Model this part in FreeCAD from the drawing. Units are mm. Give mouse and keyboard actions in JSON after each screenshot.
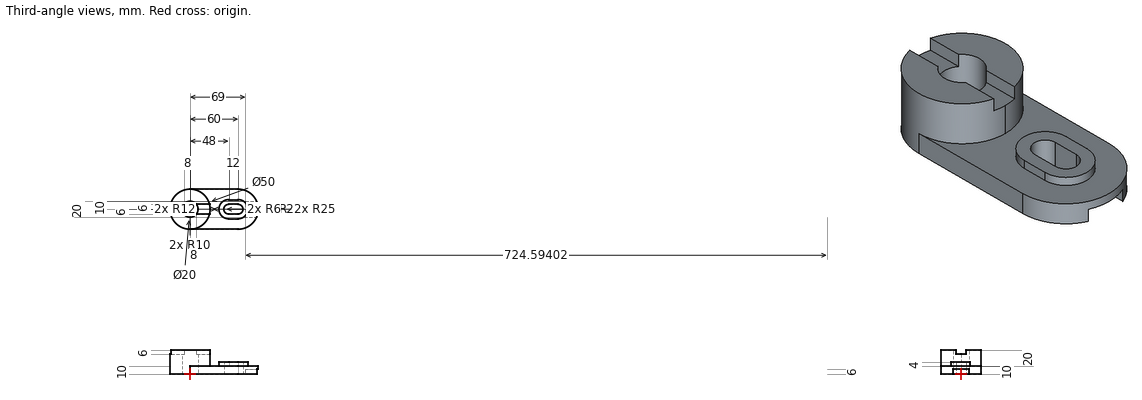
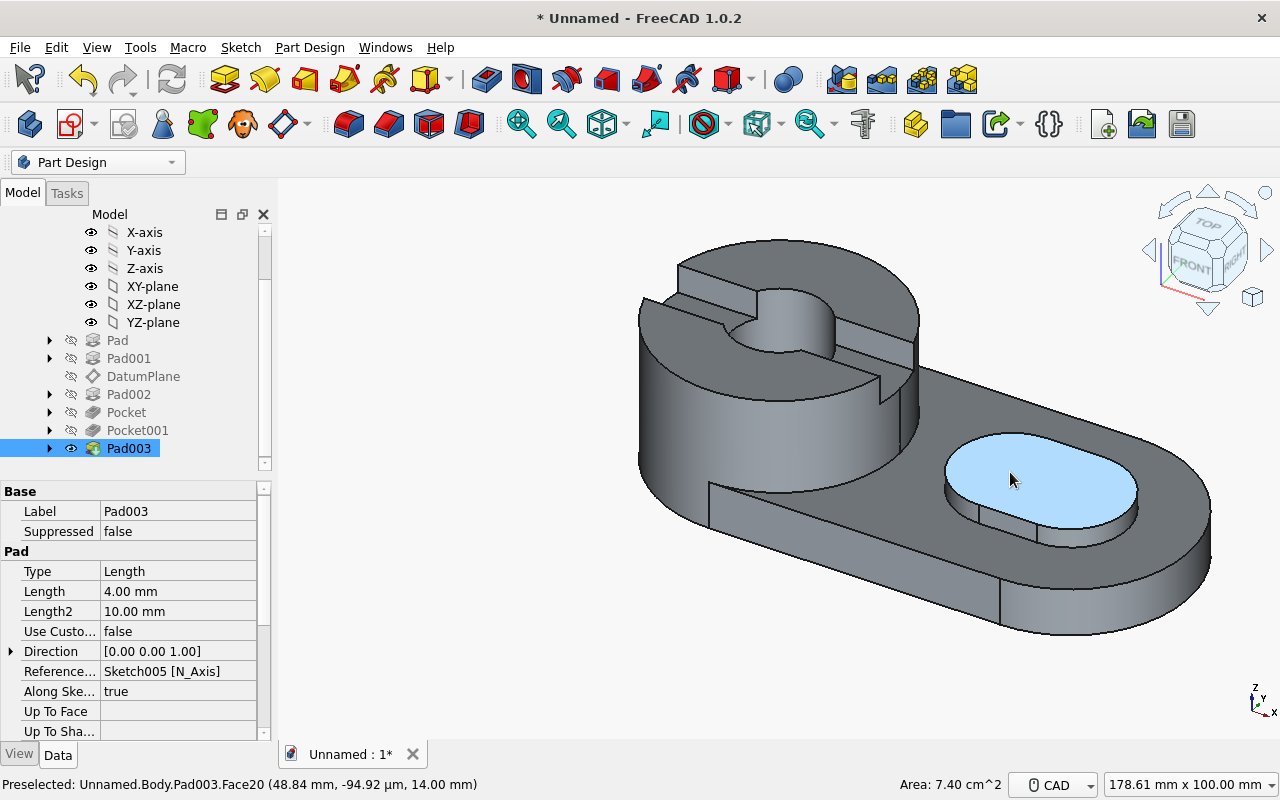
{"action": "left_click", "coordinate": [70, 124]}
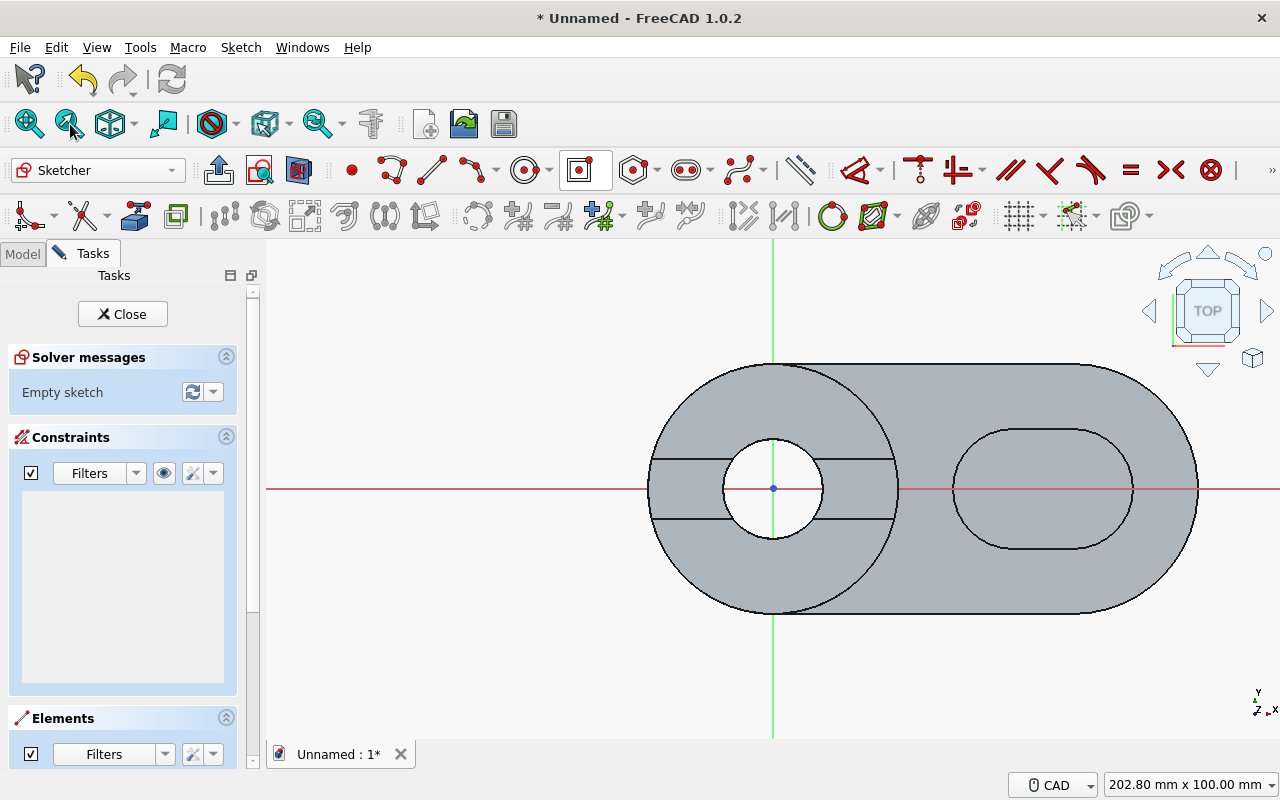
{"action": "left_click", "coordinate": [300, 170]}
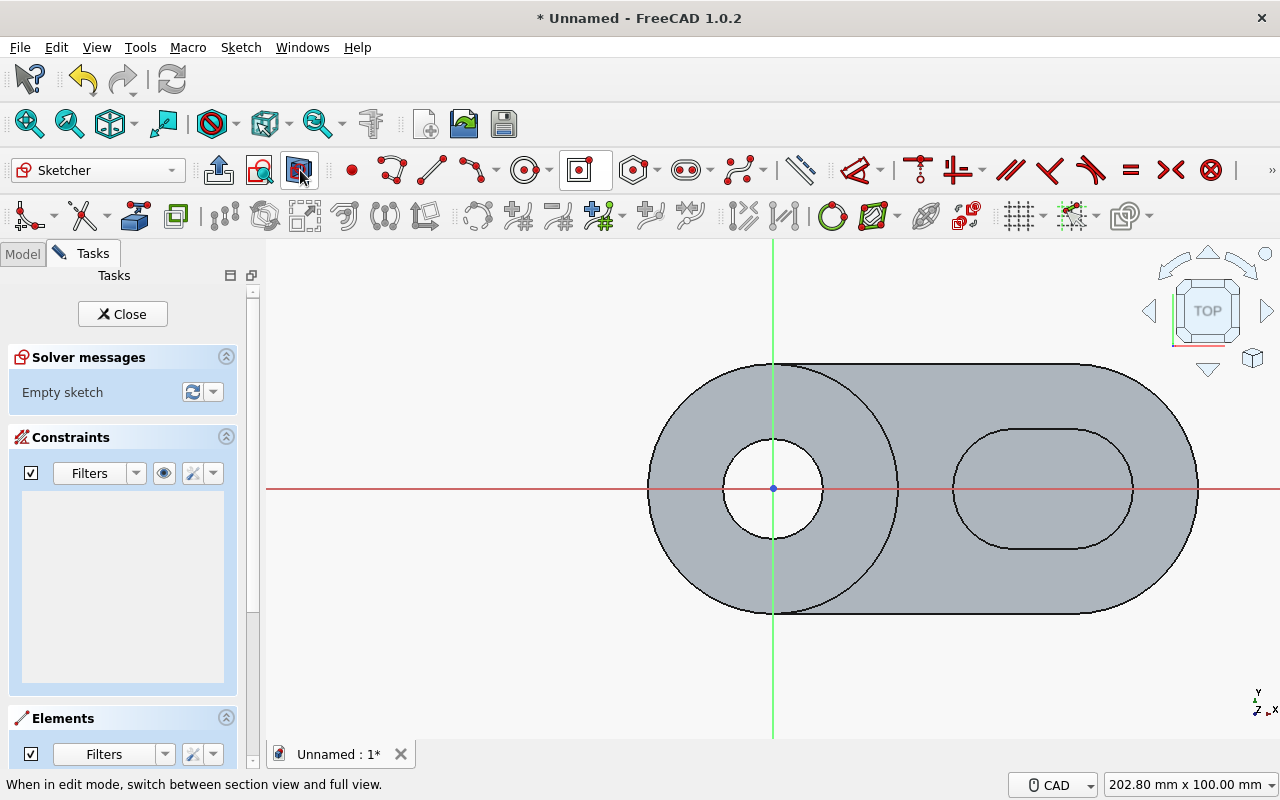
{"action": "scroll", "coordinate": [1115, 489], "scroll_direction": "up", "scroll_amount": 8}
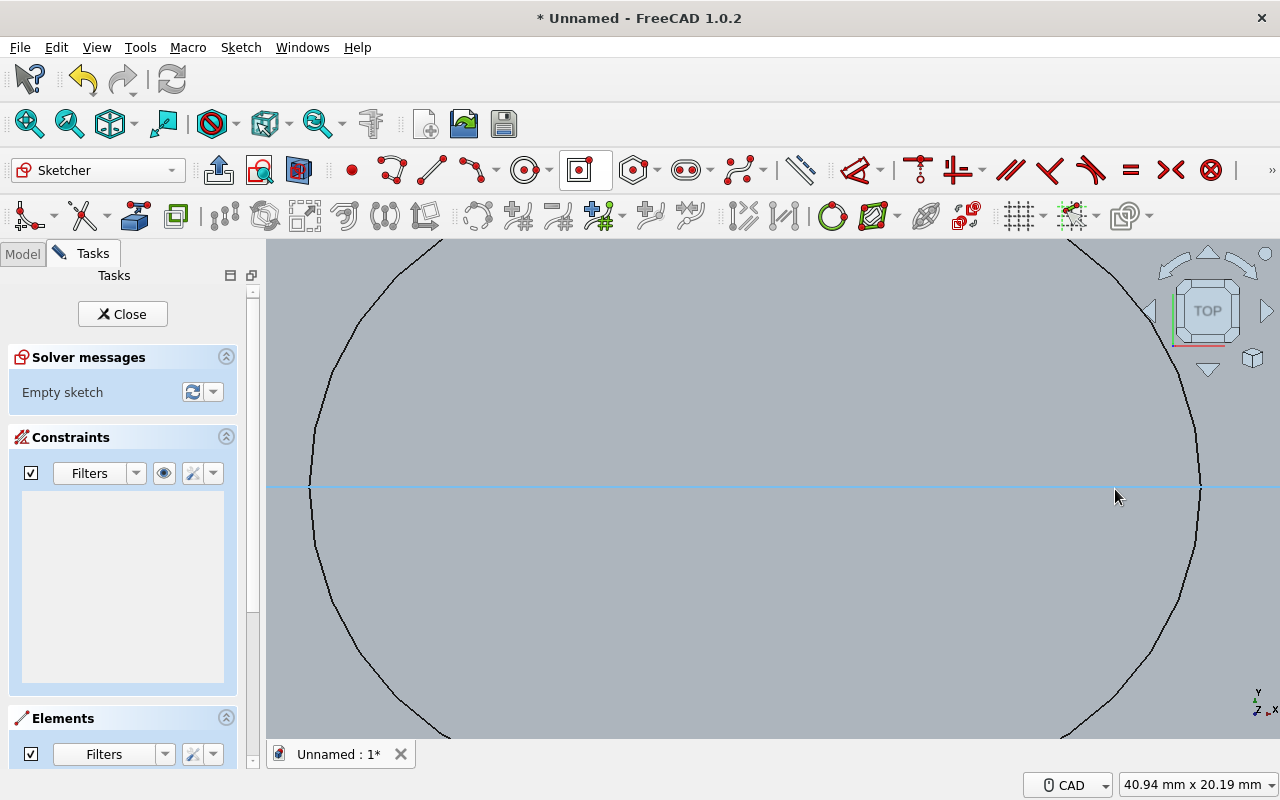
{"action": "left_click", "coordinate": [686, 170]}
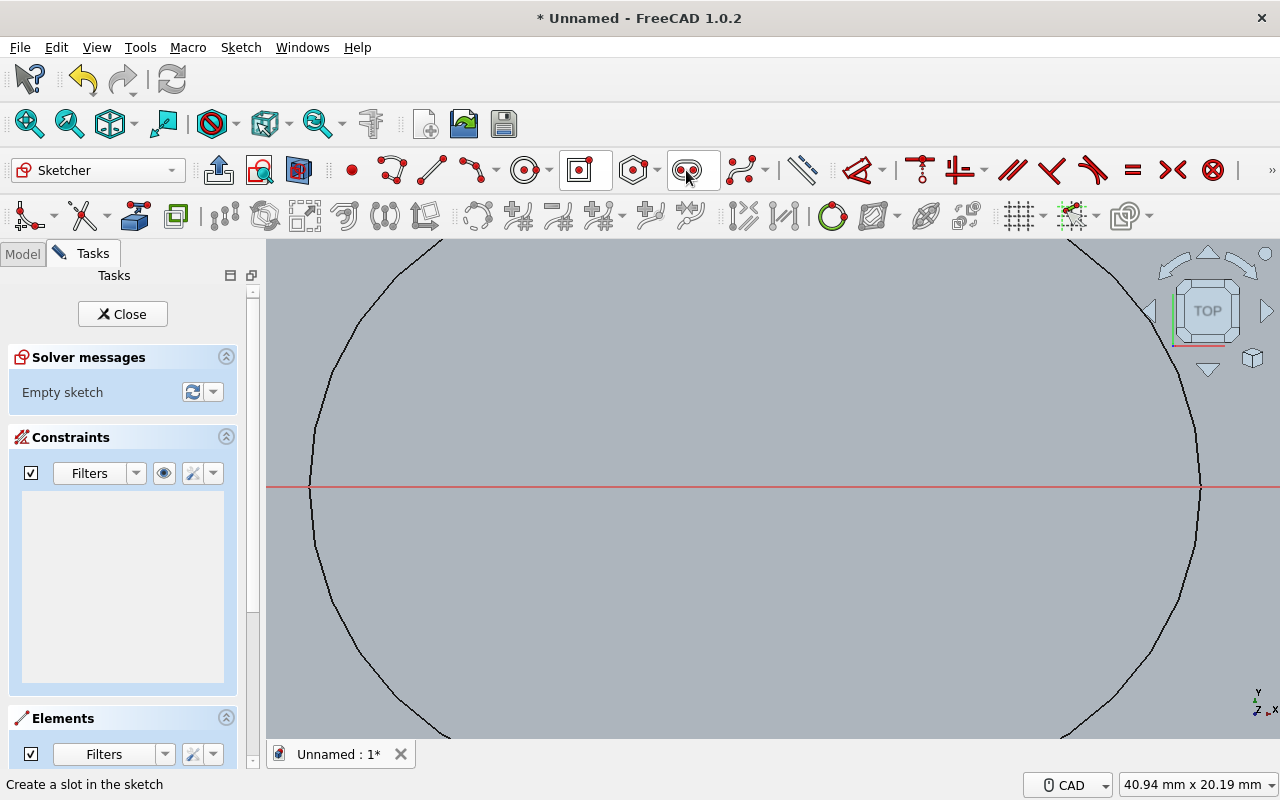
{"action": "left_click", "coordinate": [606, 487]}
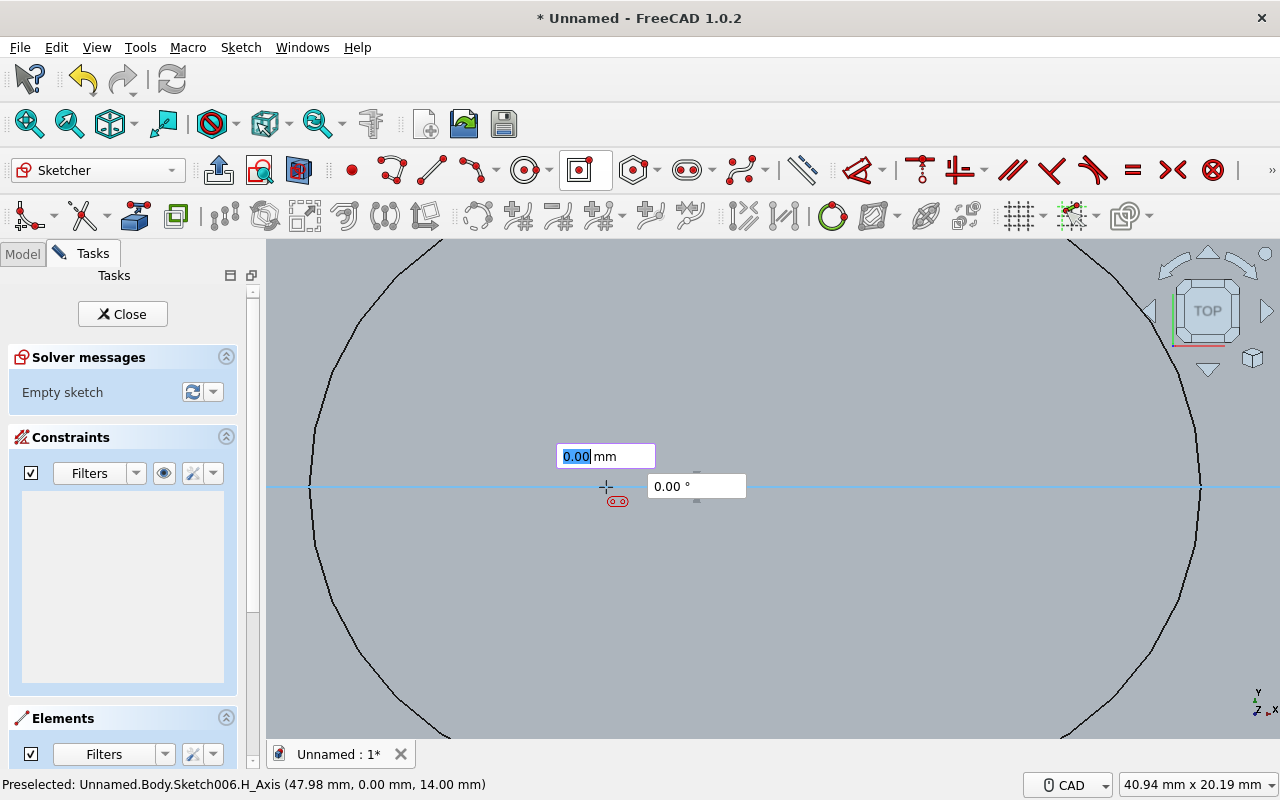
{"action": "left_click", "coordinate": [904, 478]}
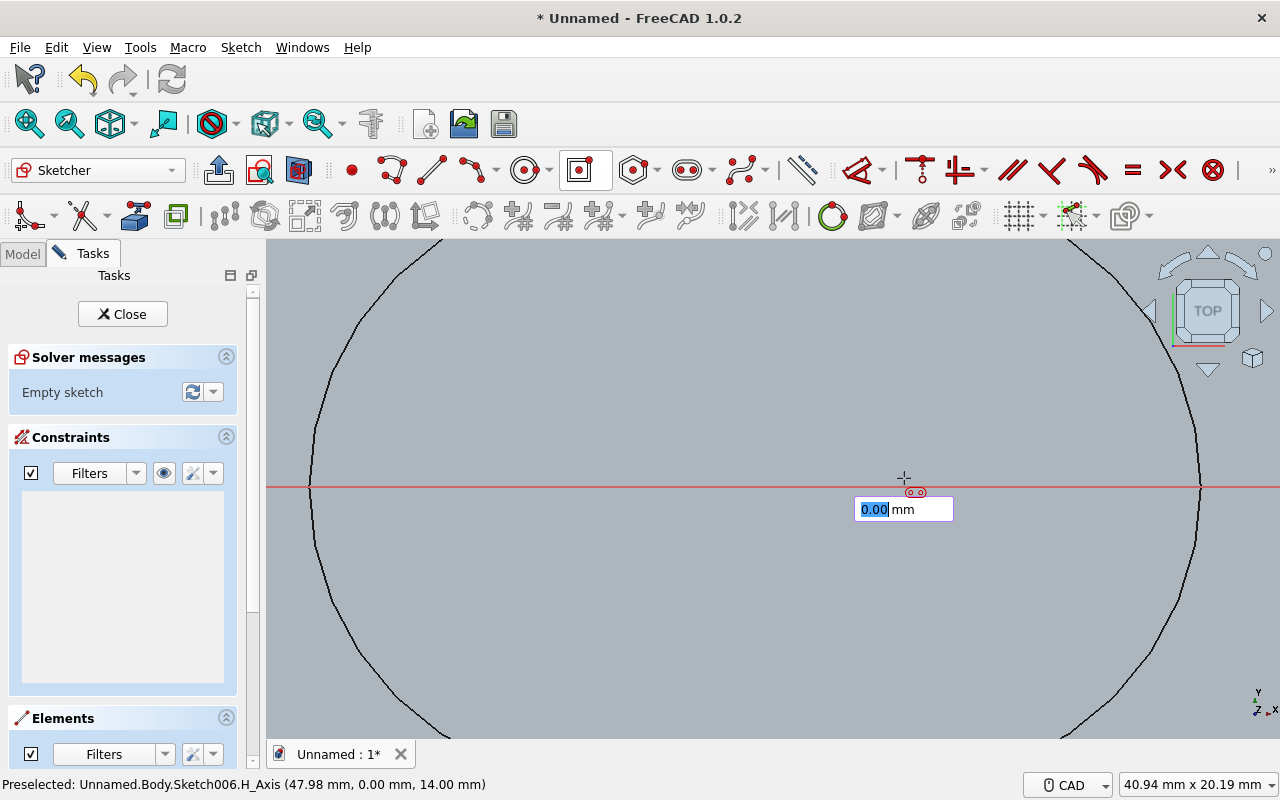
{"action": "left_click", "coordinate": [755, 338]}
{"action": "key", "text": "Escape"}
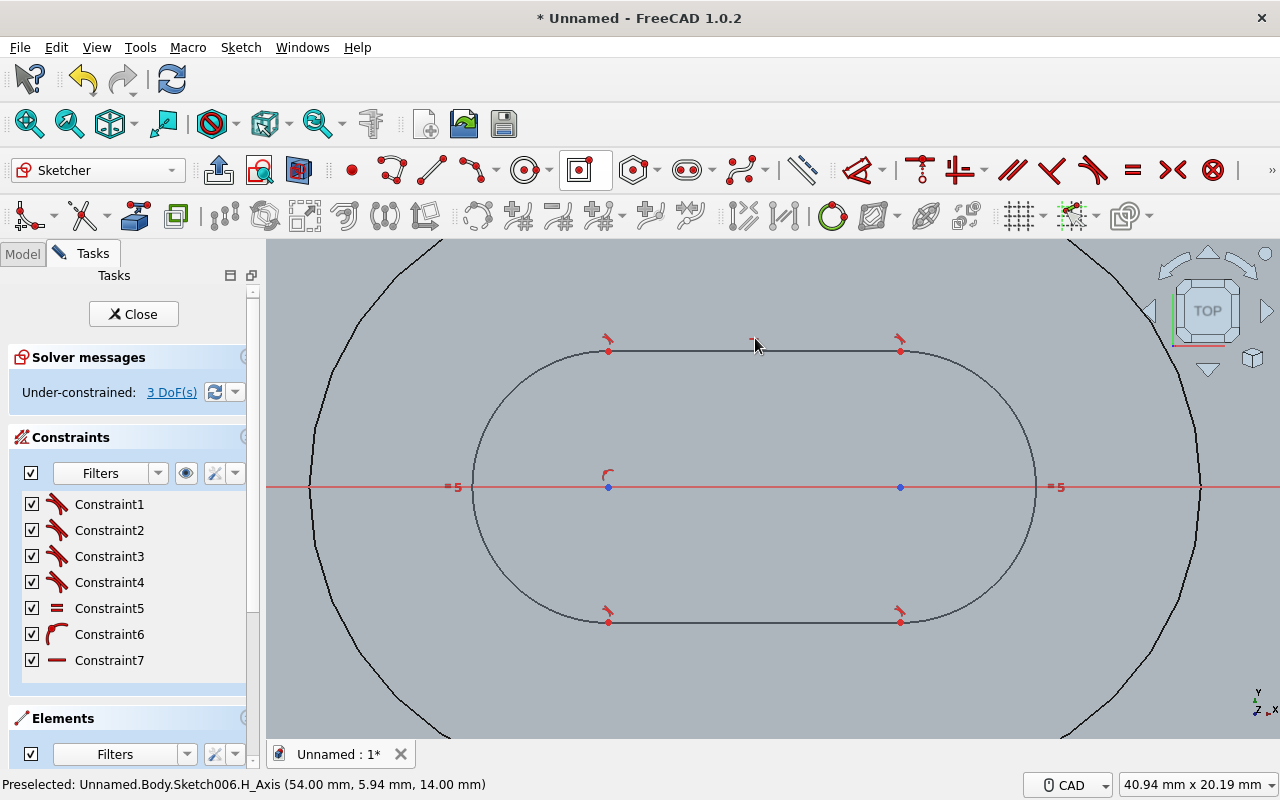
{"action": "left_click", "coordinate": [858, 170]}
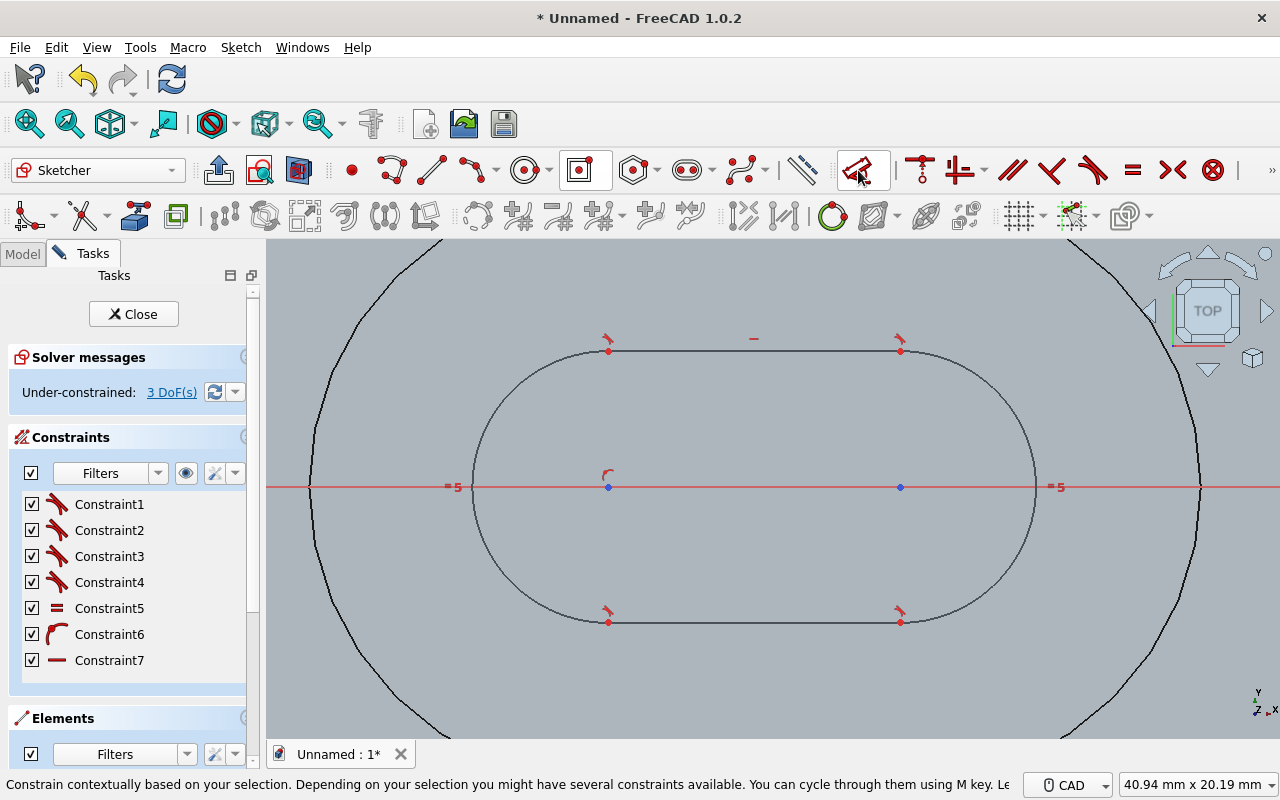
{"action": "left_click", "coordinate": [498, 407]}
{"action": "left_click", "coordinate": [472, 388]}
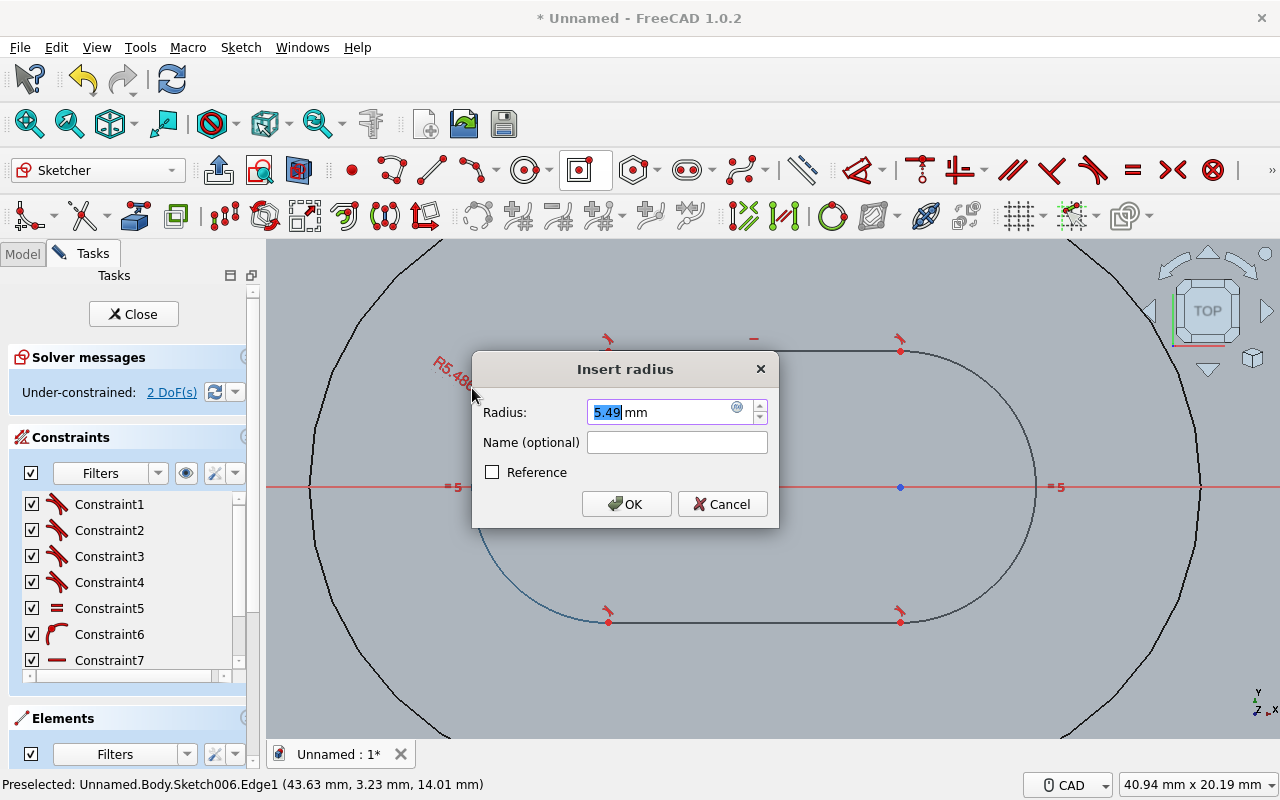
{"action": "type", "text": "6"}
{"action": "key", "text": "Return"}